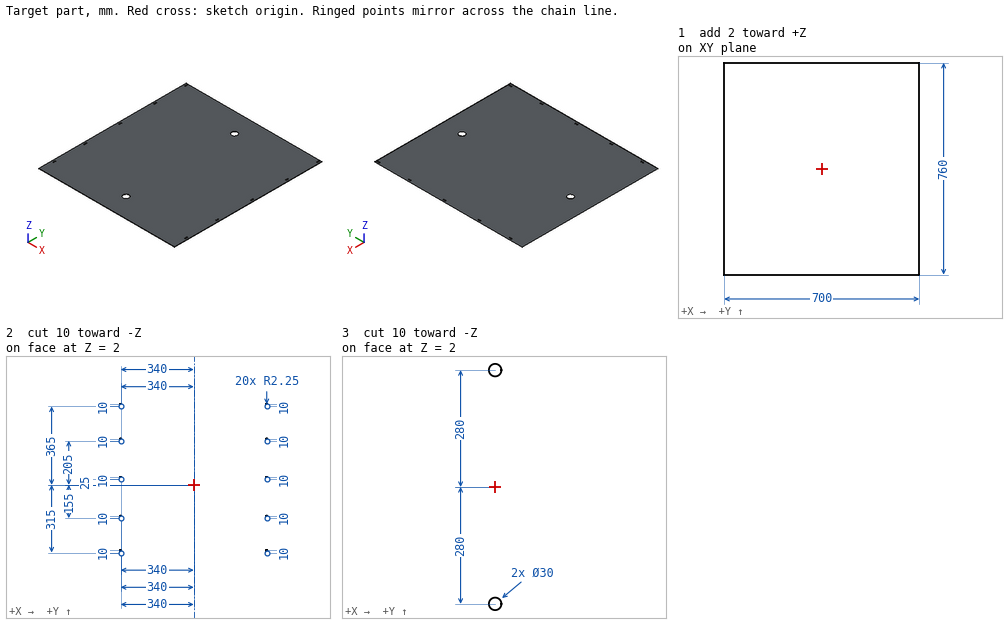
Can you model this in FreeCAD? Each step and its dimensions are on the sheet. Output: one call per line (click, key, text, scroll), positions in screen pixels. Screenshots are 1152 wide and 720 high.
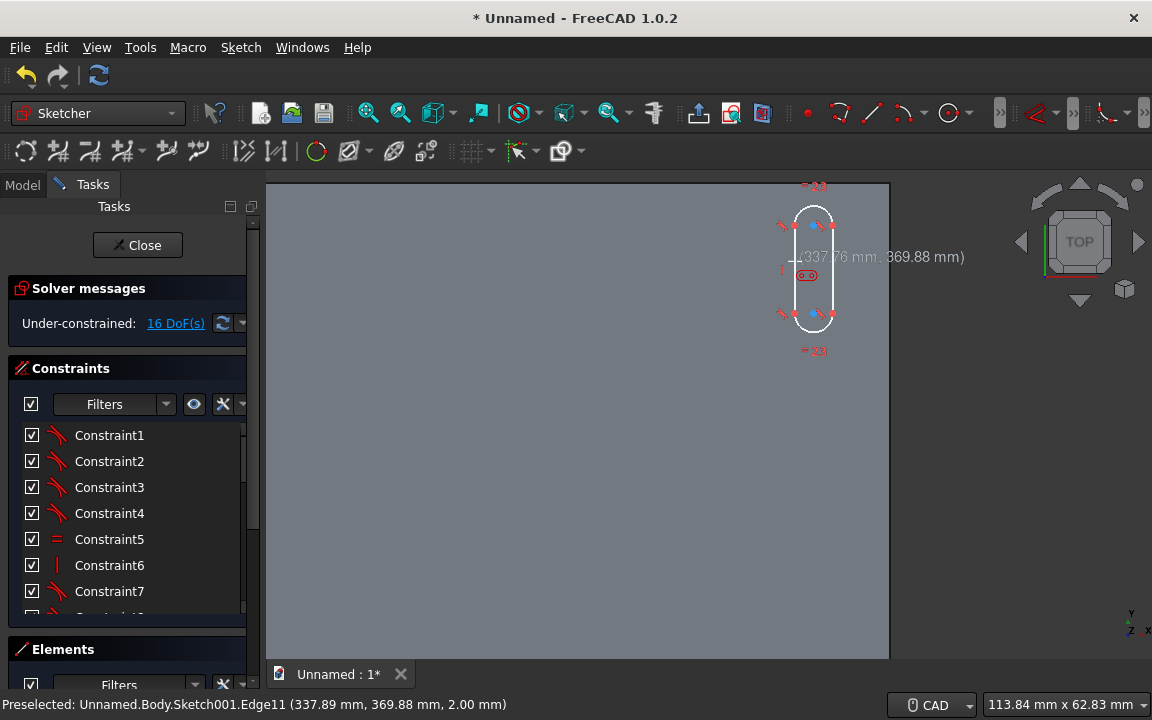
scroll(801, 253, down, 14)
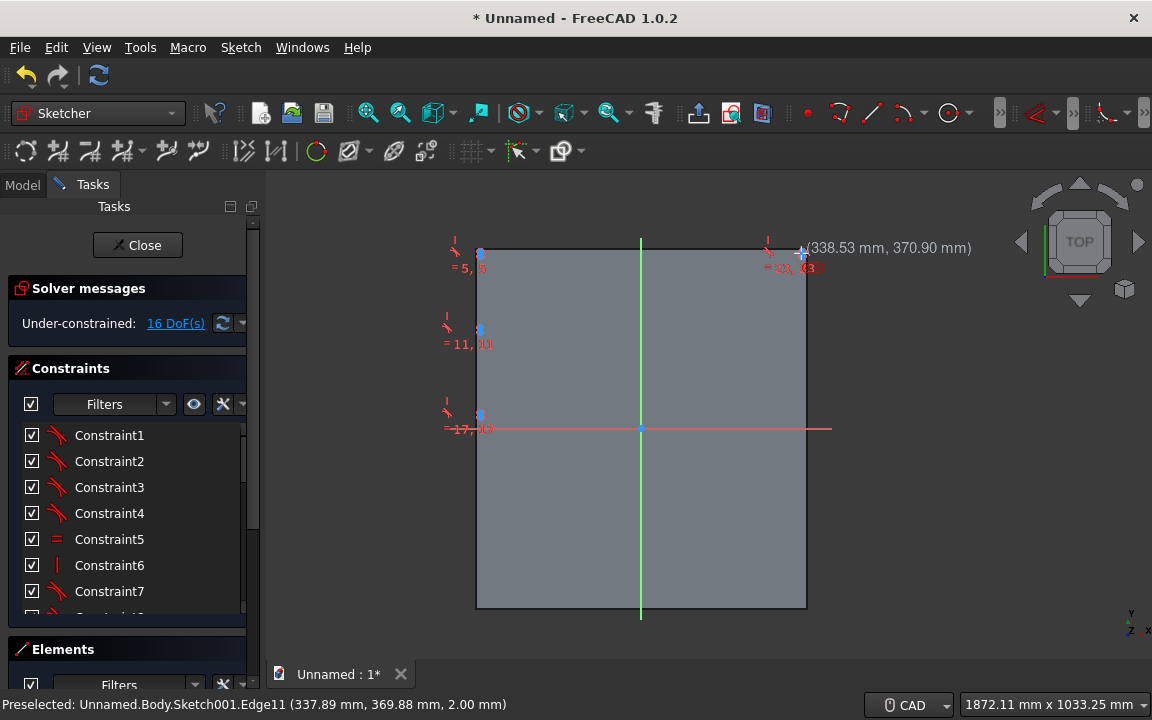
scroll(802, 332, up, 16)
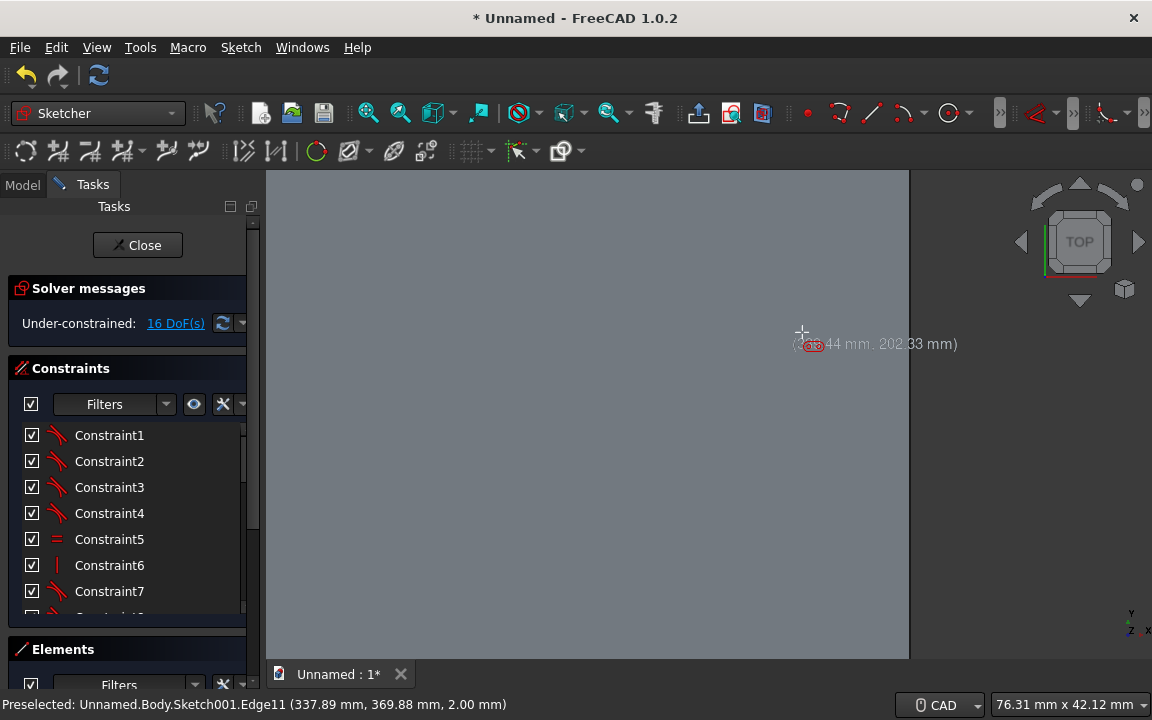
scroll(802, 332, down, 16)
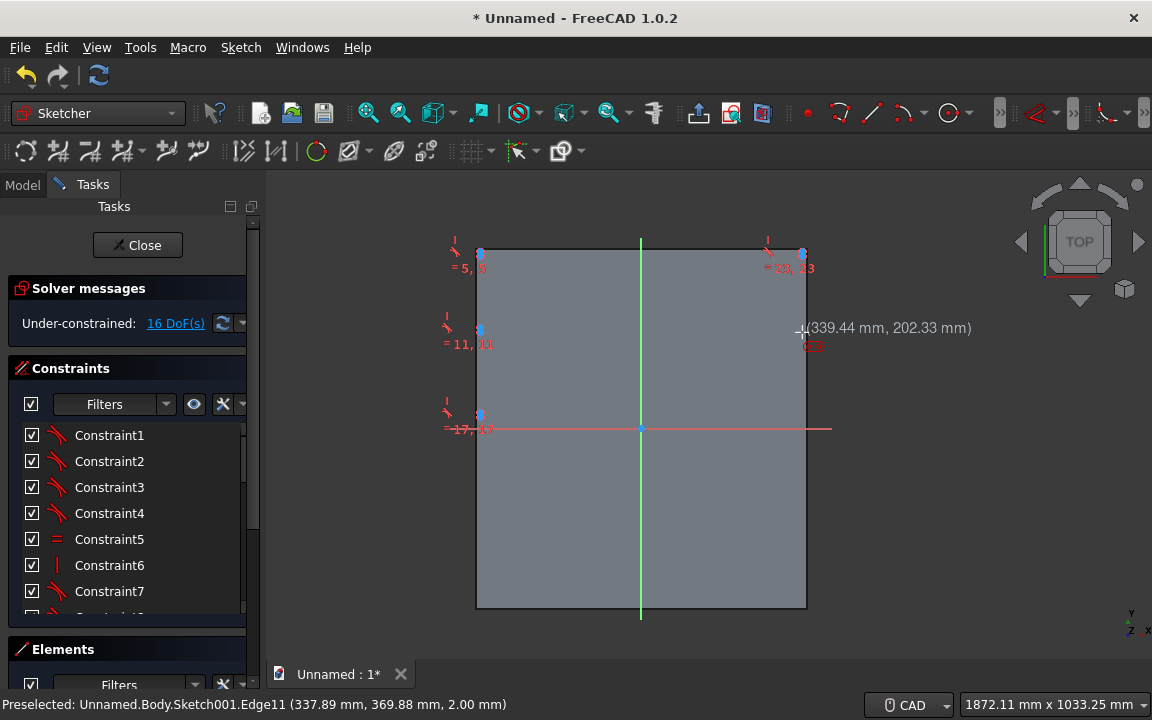
click(802, 332)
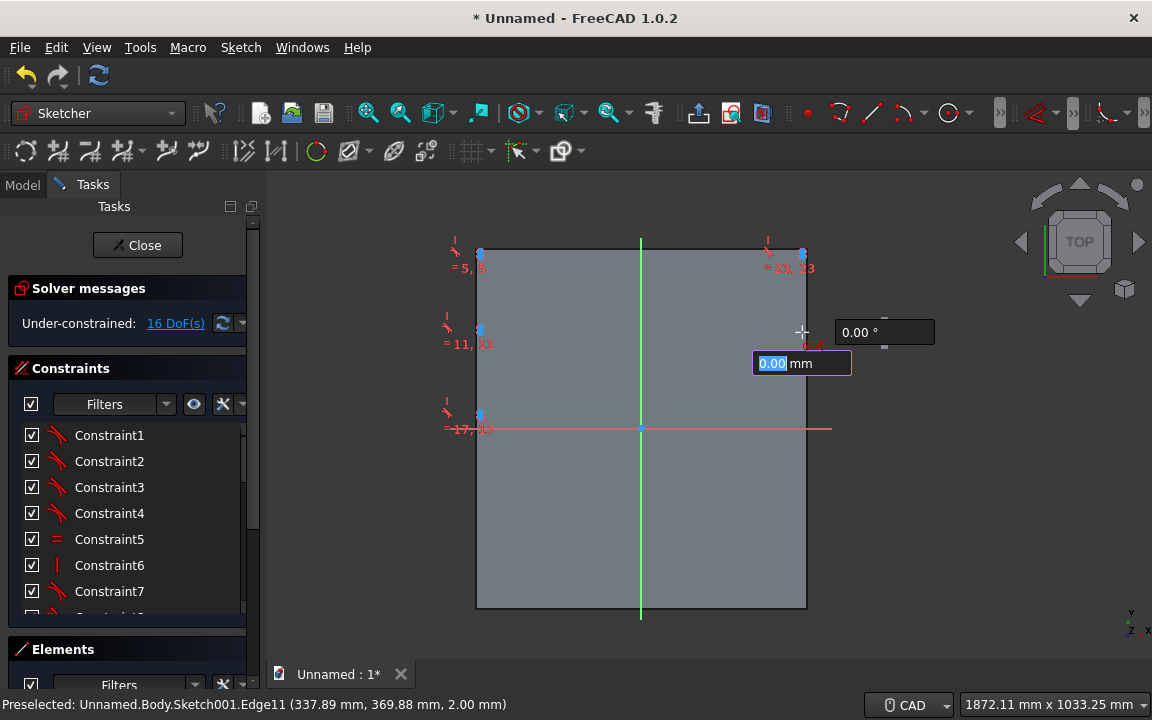
scroll(802, 327, up, 7)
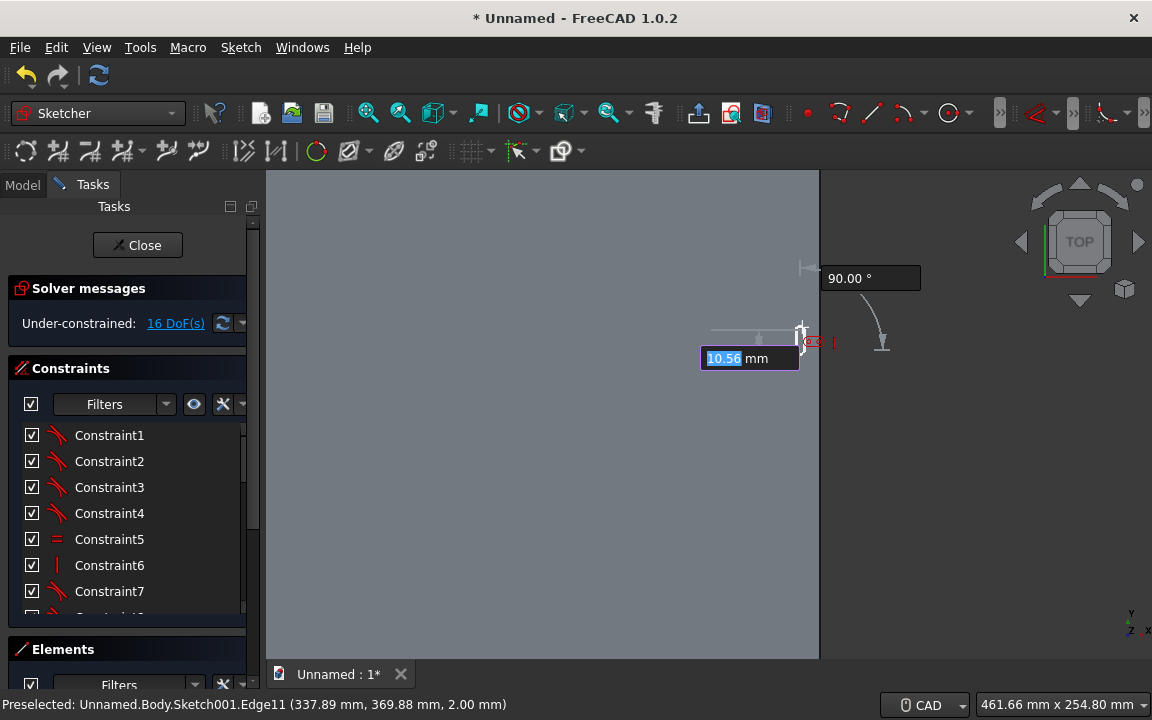
click(800, 326)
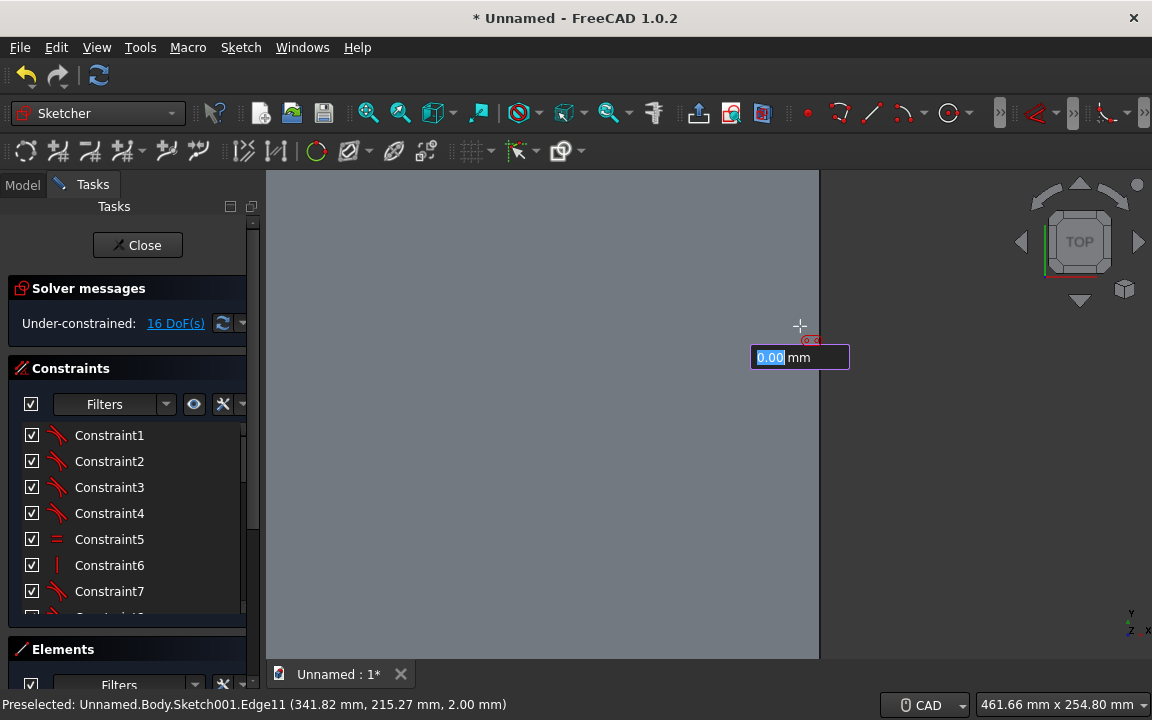
scroll(806, 336, up, 7)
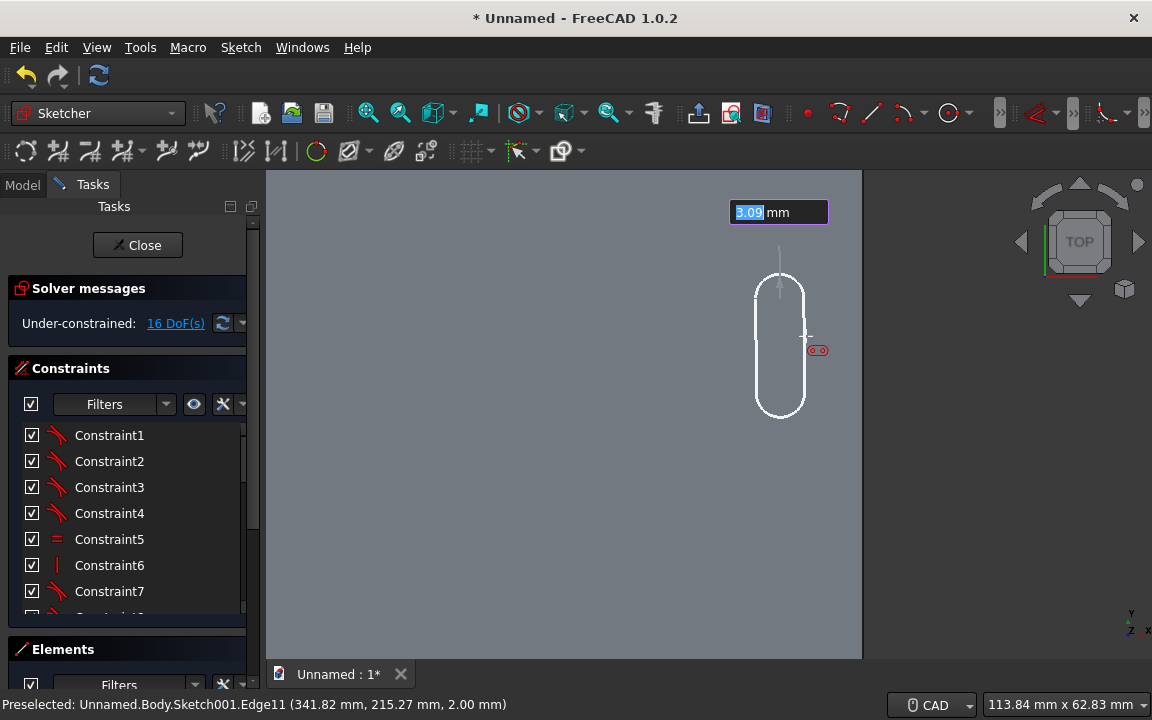
click(802, 333)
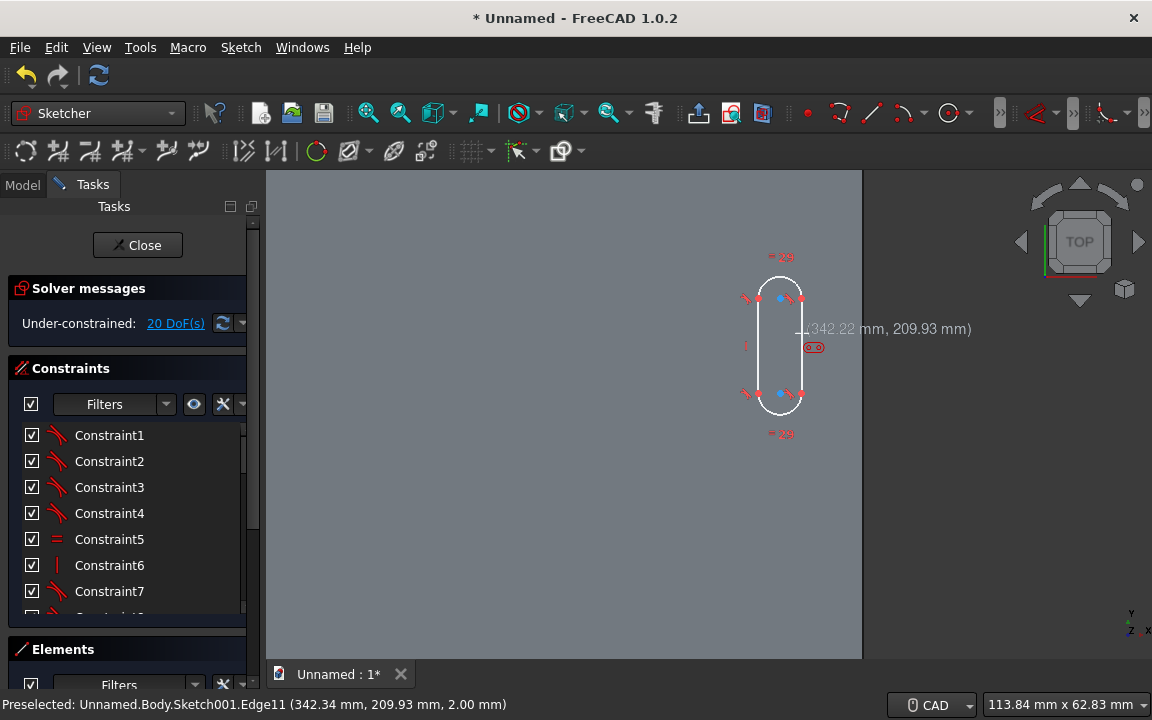
scroll(802, 329, down, 14)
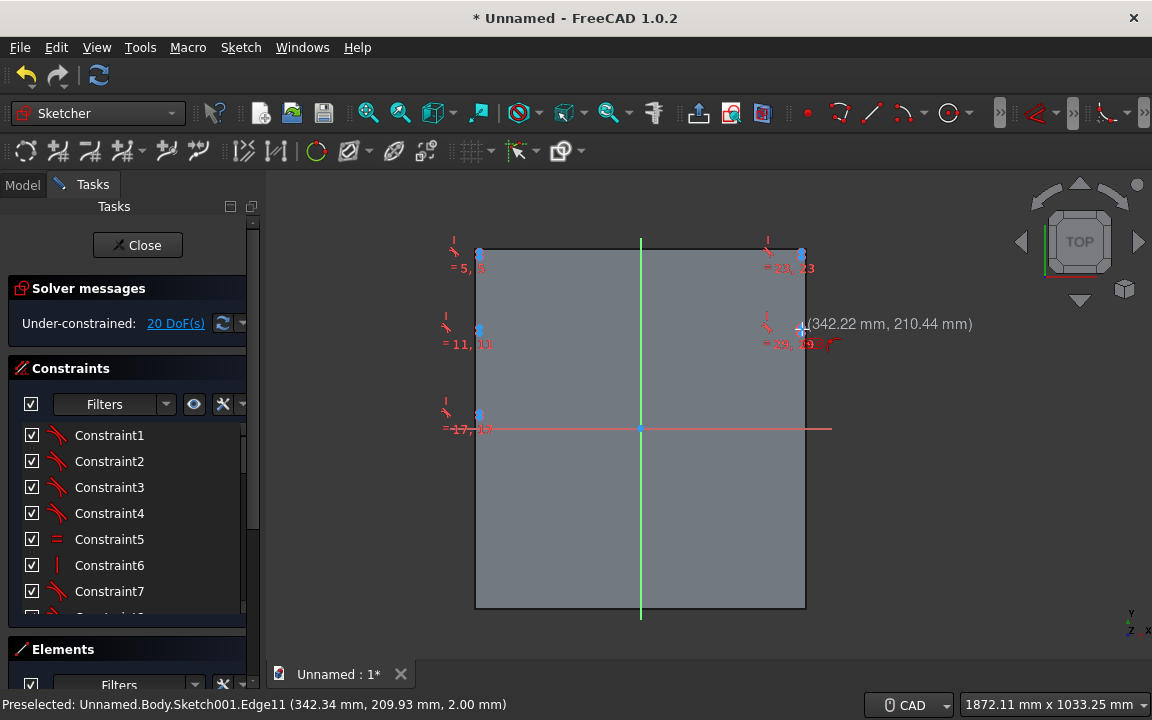
scroll(802, 417, up, 16)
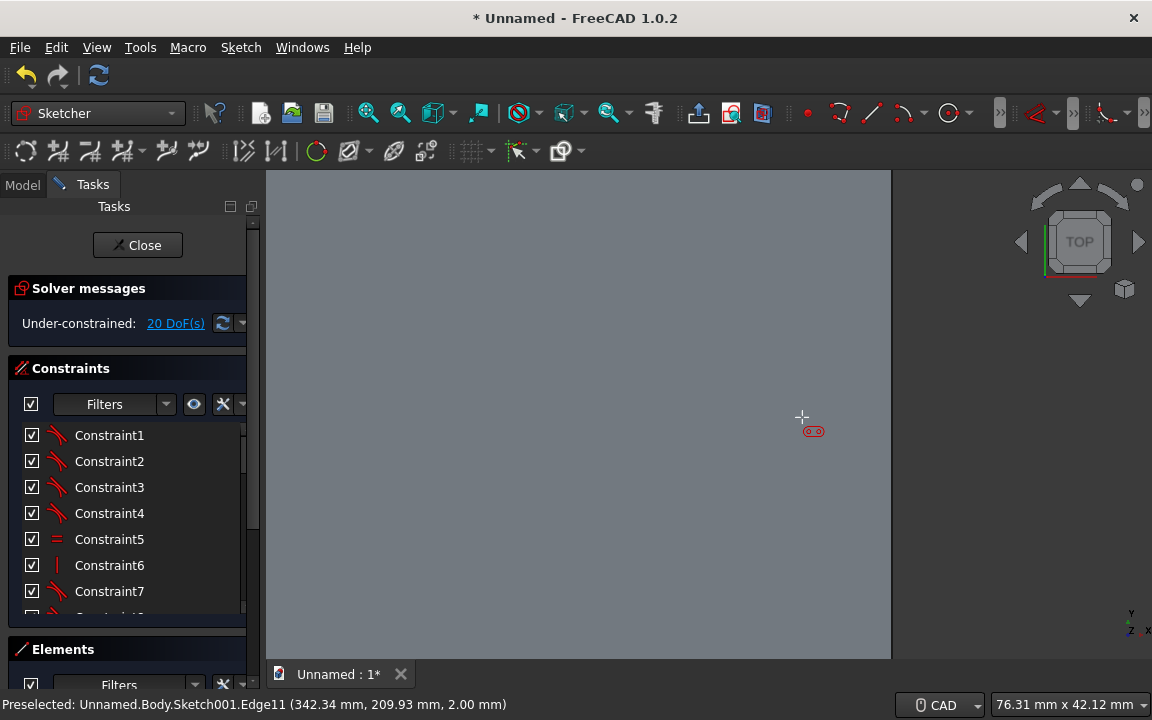
scroll(802, 417, down, 16)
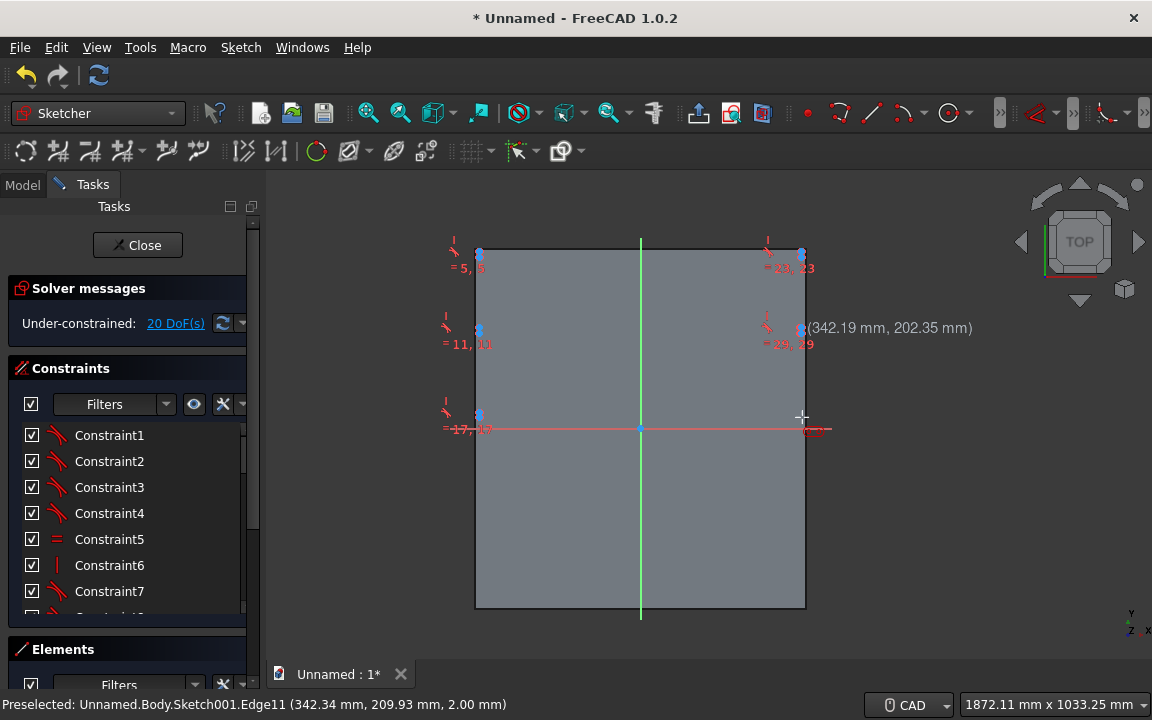
scroll(802, 417, up, 2)